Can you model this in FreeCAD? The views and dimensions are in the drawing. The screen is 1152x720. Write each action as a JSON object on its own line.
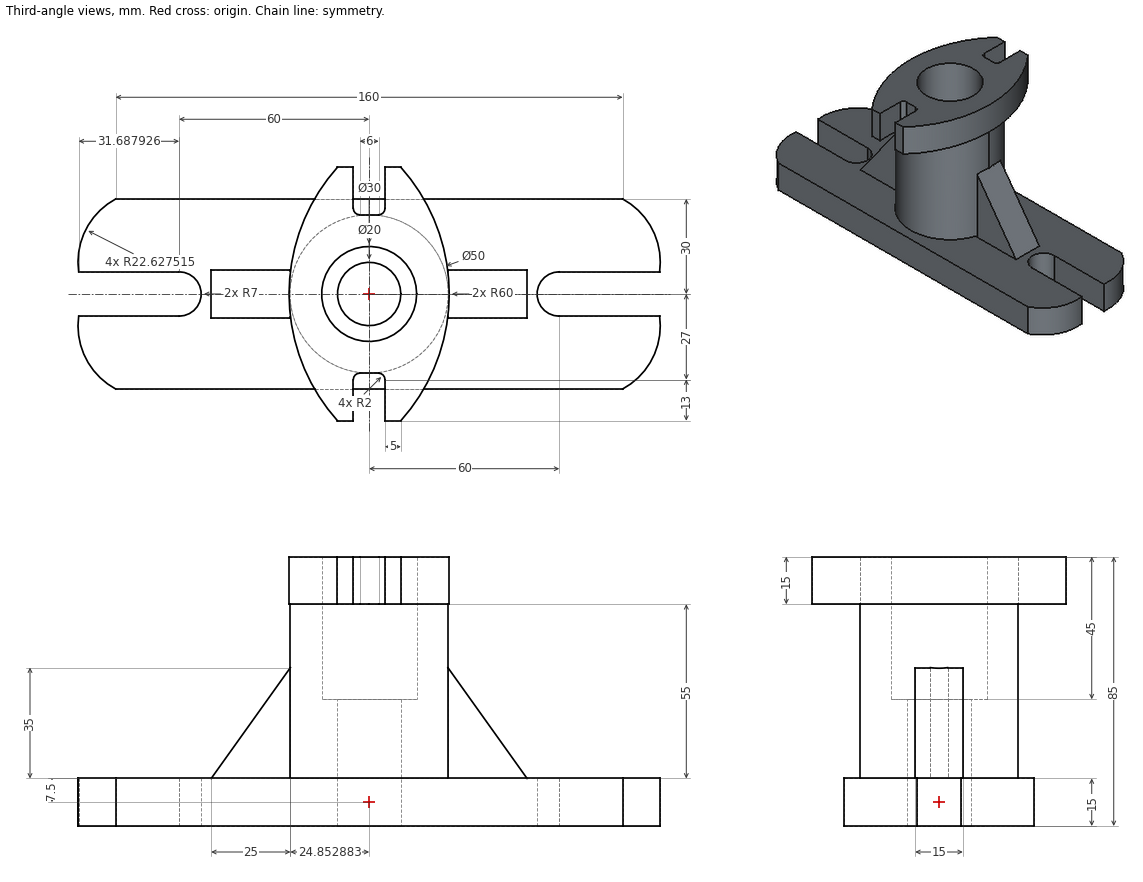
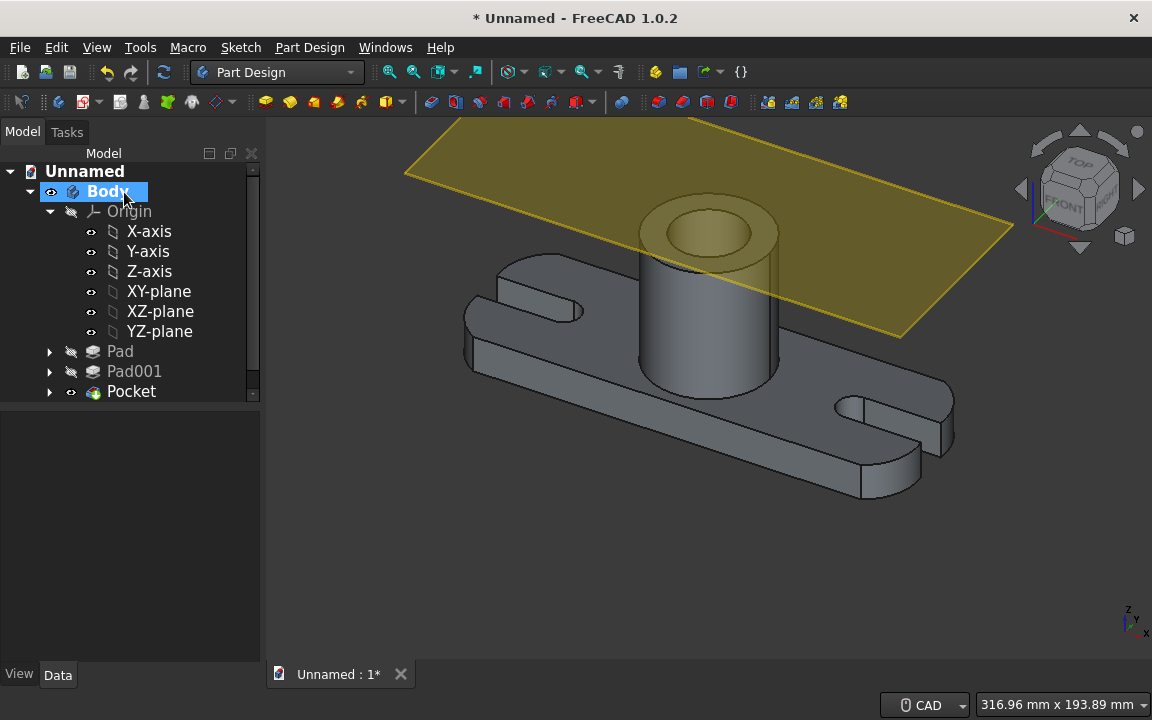
{"action": "scroll", "coordinate": [100, 287], "scroll_direction": "down", "scroll_amount": 3}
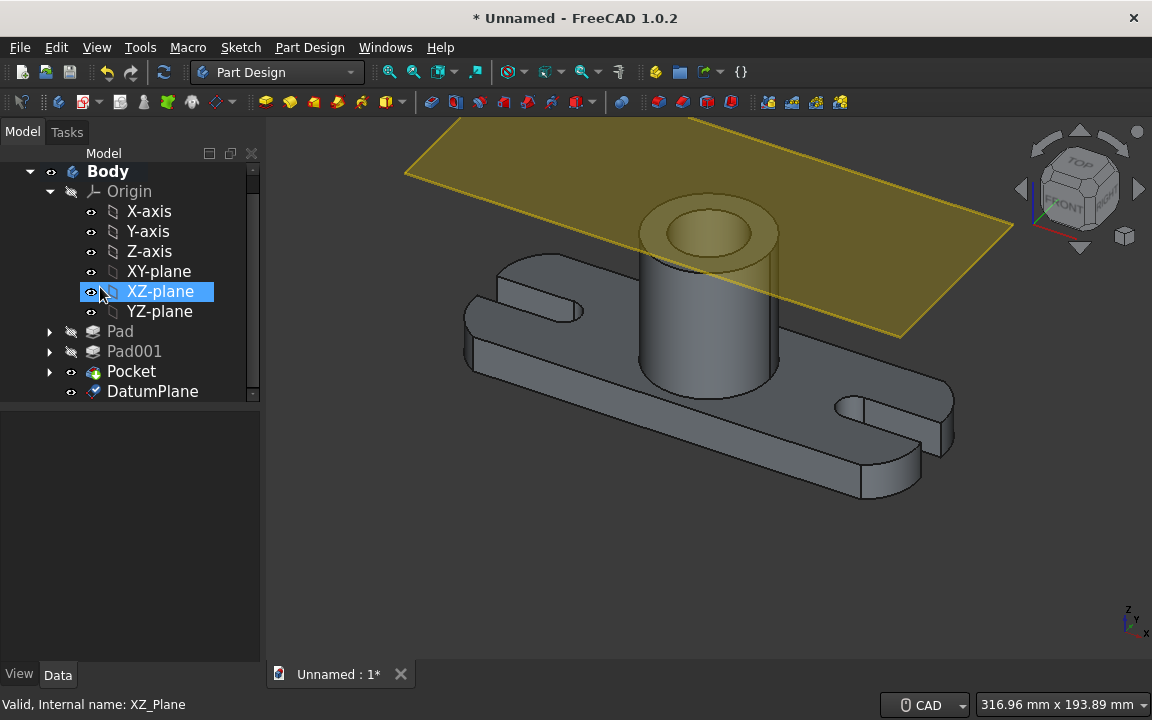
{"action": "left_click", "coordinate": [116, 392]}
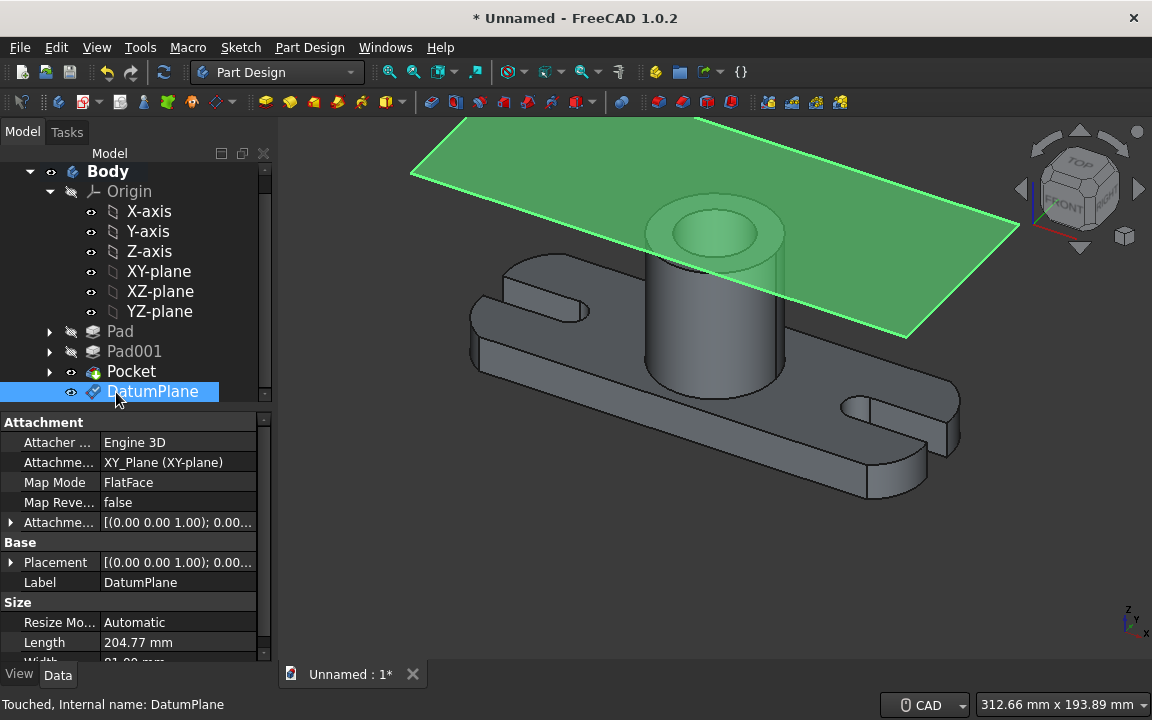
{"action": "left_click", "coordinate": [84, 102]}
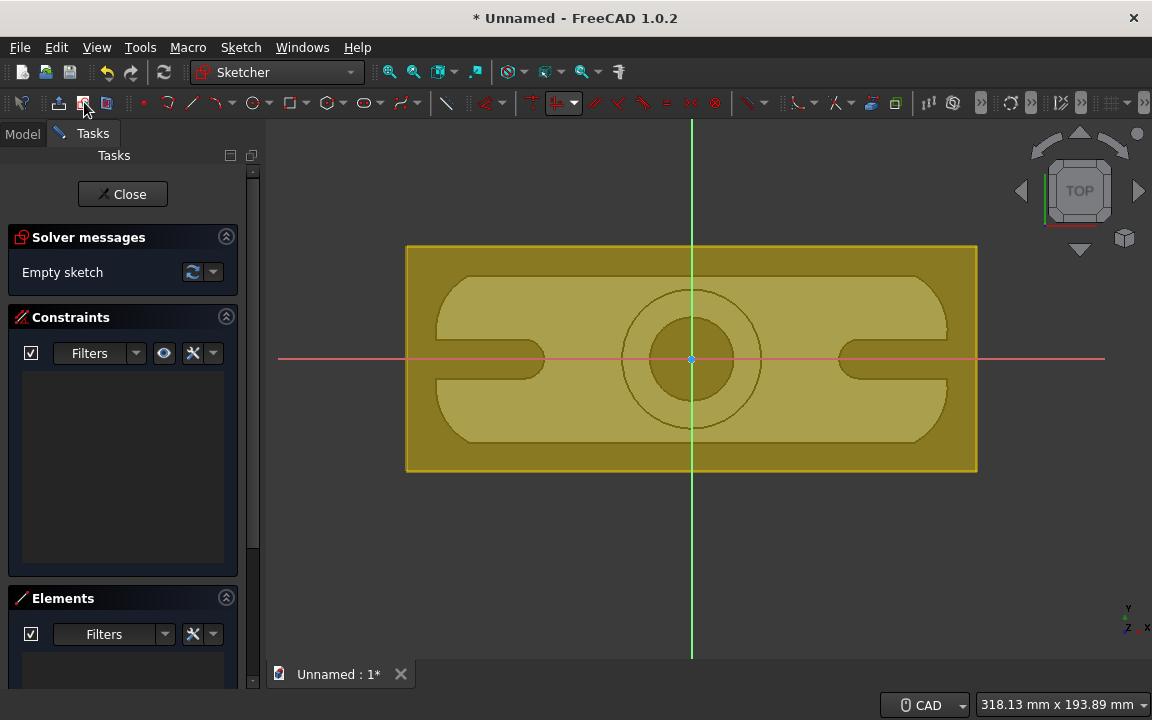
{"action": "scroll", "coordinate": [796, 298], "scroll_direction": "up", "scroll_amount": 2}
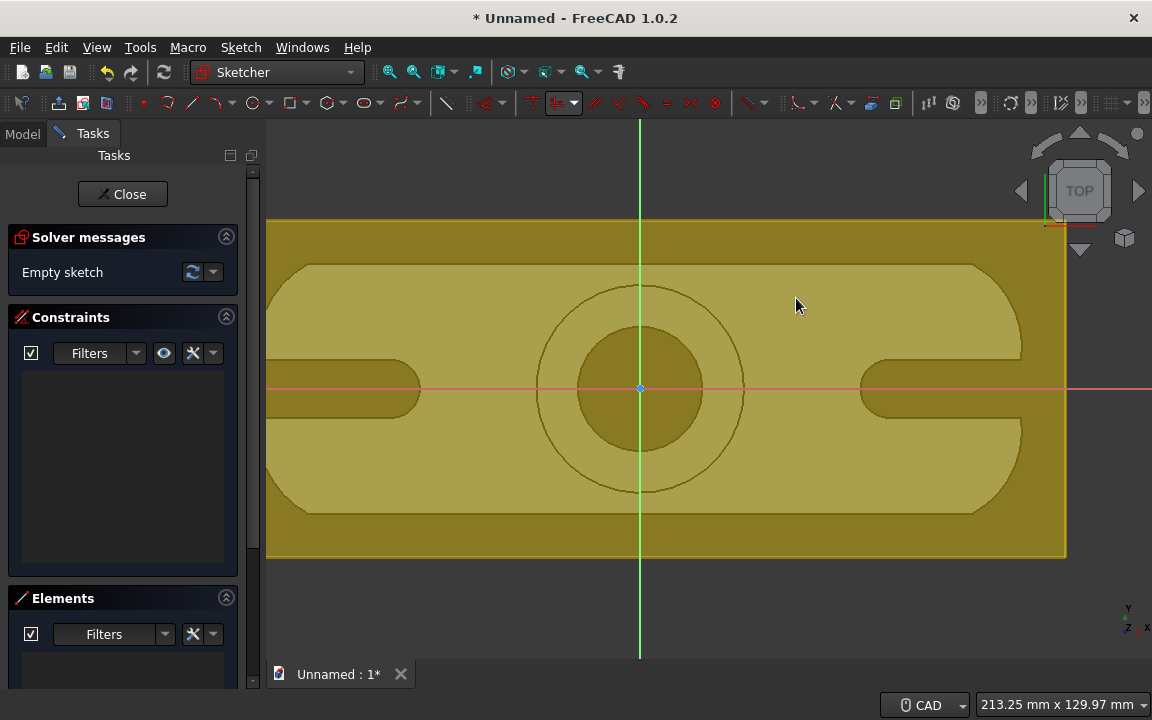
{"action": "left_click", "coordinate": [168, 104]}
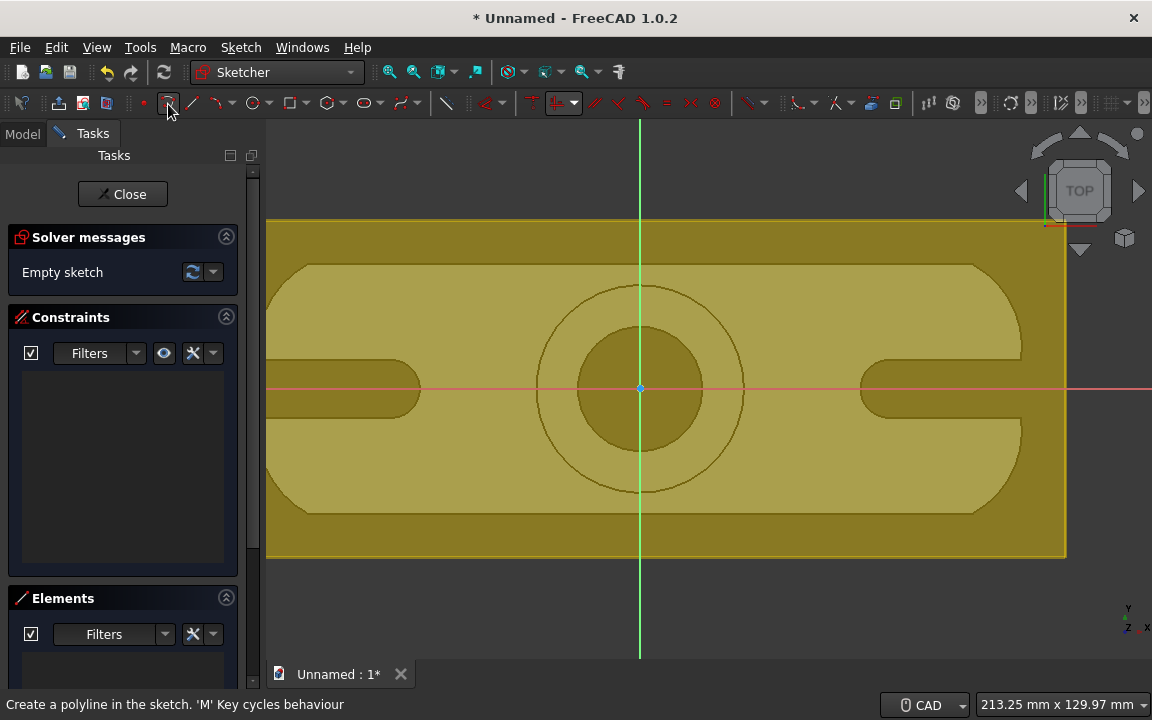
{"action": "left_click", "coordinate": [661, 501]}
{"action": "left_click", "coordinate": [661, 555]}
{"action": "left_click", "coordinate": [682, 555]}
{"action": "right_click", "coordinate": [682, 555]}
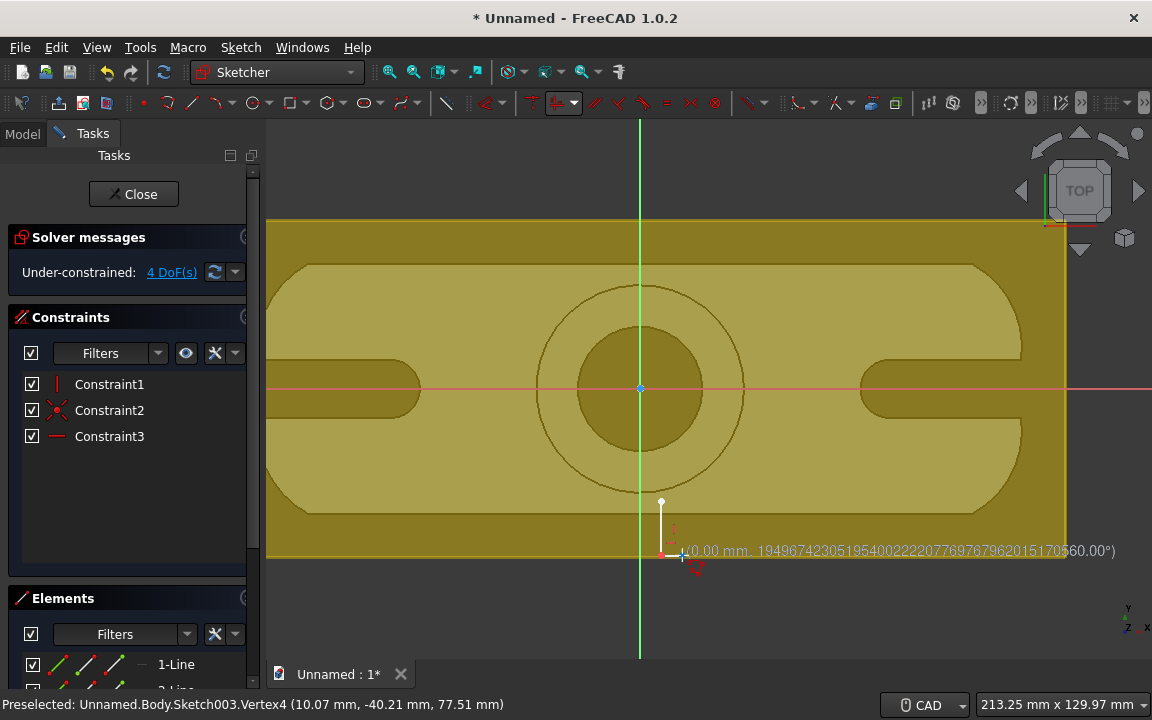
{"action": "left_click", "coordinate": [682, 223]}
{"action": "left_click", "coordinate": [661, 223]}
{"action": "left_click", "coordinate": [661, 277]}
{"action": "right_click", "coordinate": [661, 277]}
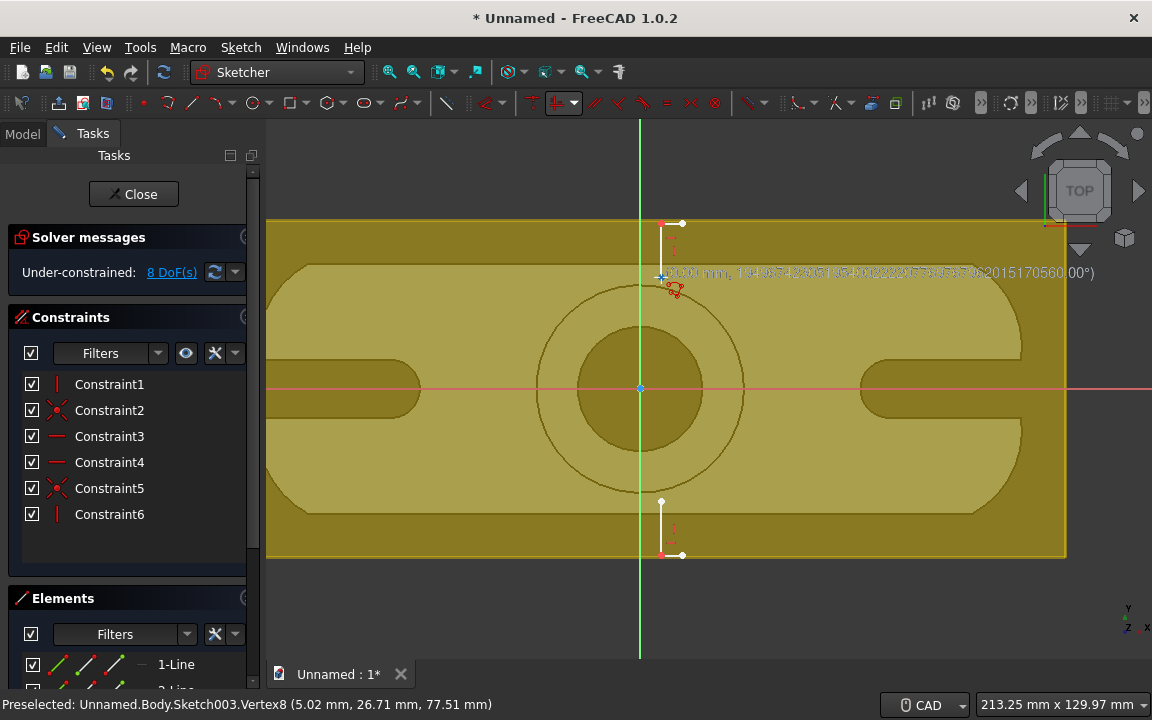
{"action": "key", "text": "g l"}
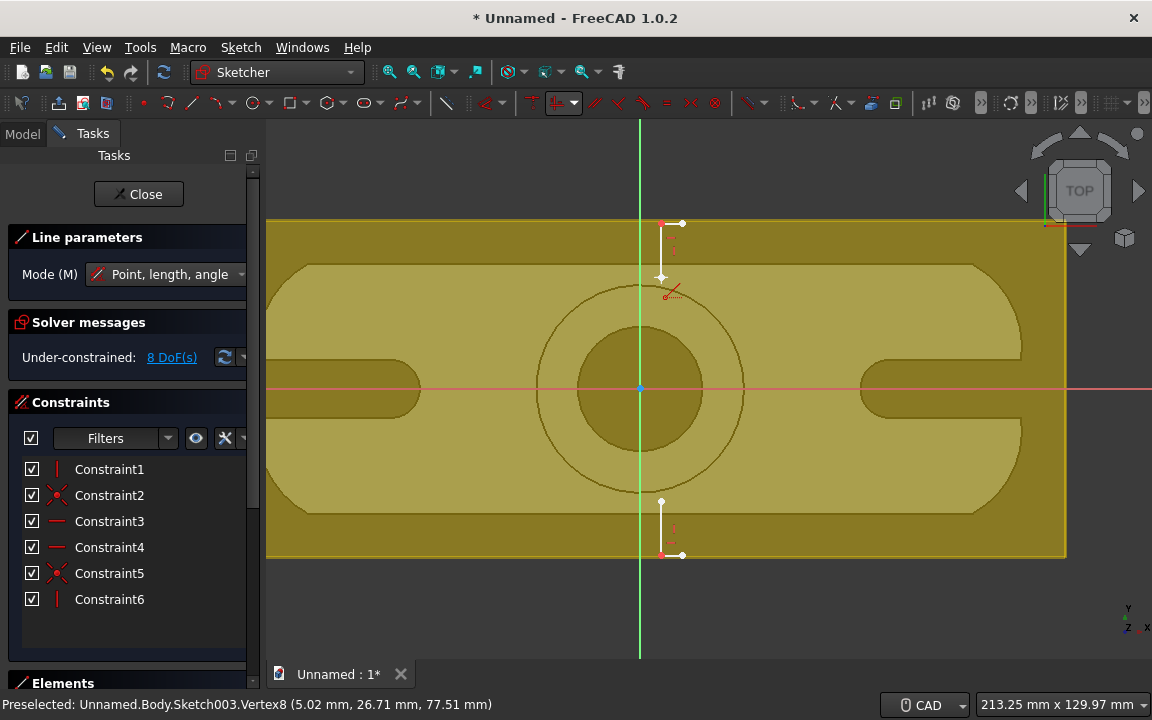
{"action": "scroll", "coordinate": [653, 285], "scroll_direction": "up", "scroll_amount": 2}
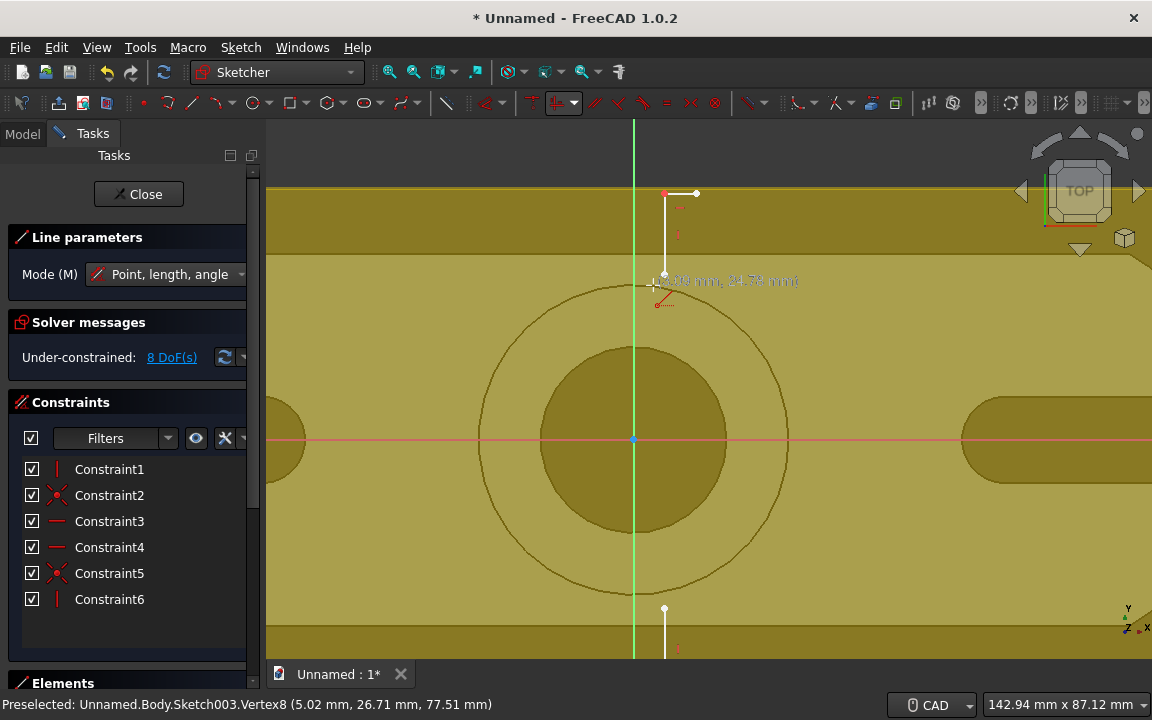
{"action": "left_click", "coordinate": [652, 285]}
{"action": "left_click", "coordinate": [615, 285]}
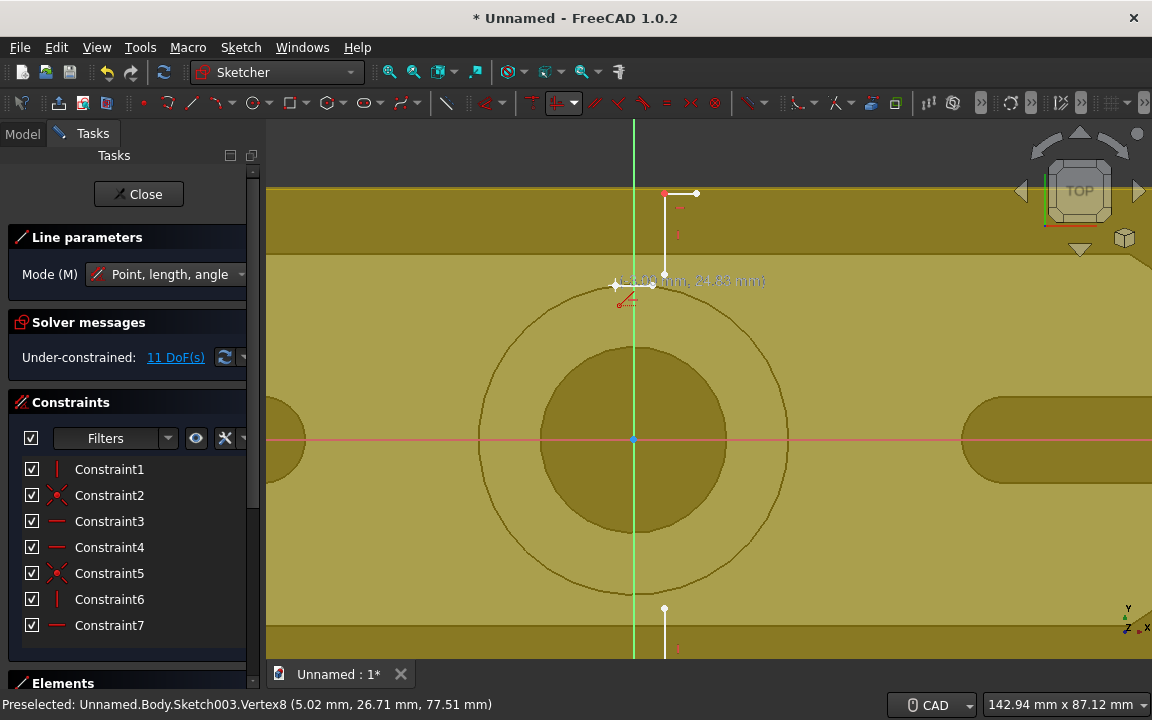
{"action": "key", "text": "g m"}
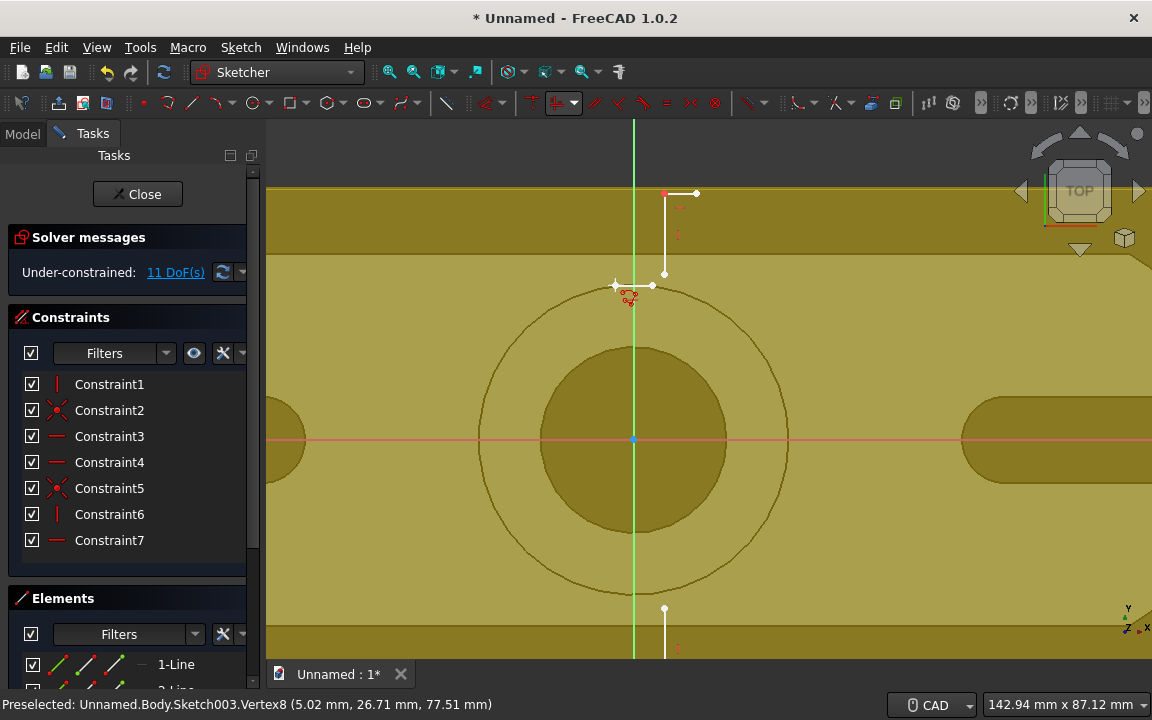
{"action": "left_click", "coordinate": [603, 273]}
{"action": "left_click", "coordinate": [603, 192]}
{"action": "left_click", "coordinate": [572, 192]}
{"action": "right_click", "coordinate": [572, 192]}